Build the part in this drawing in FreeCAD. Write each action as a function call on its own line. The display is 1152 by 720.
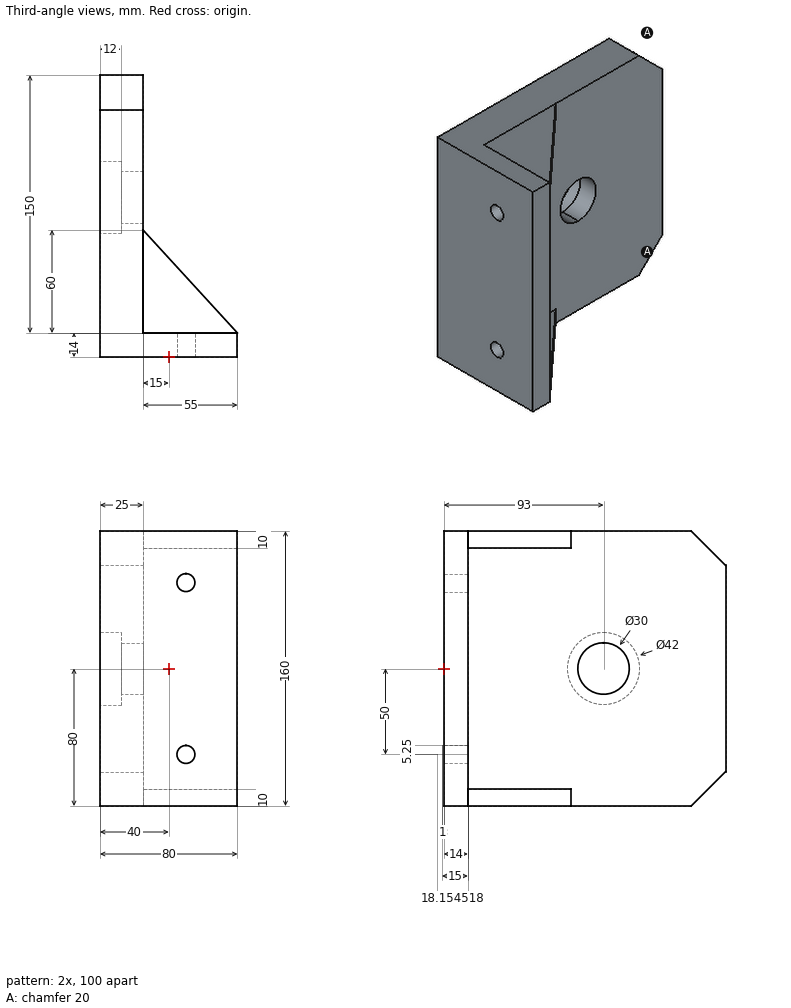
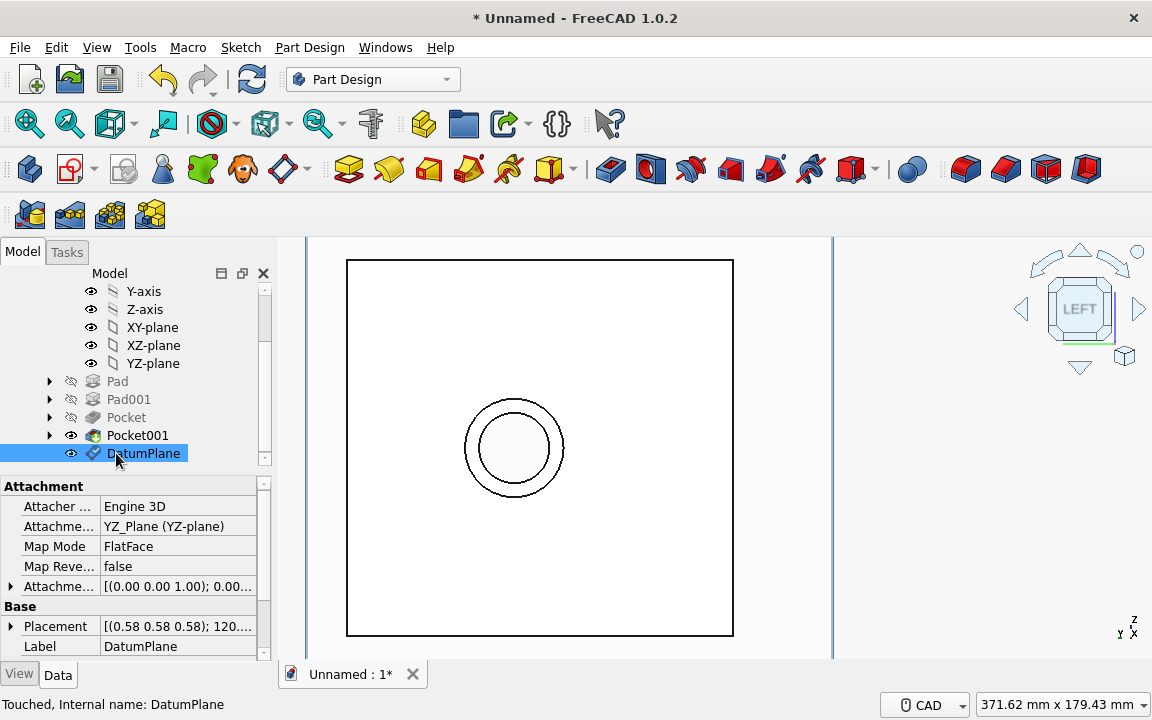
click(70, 170)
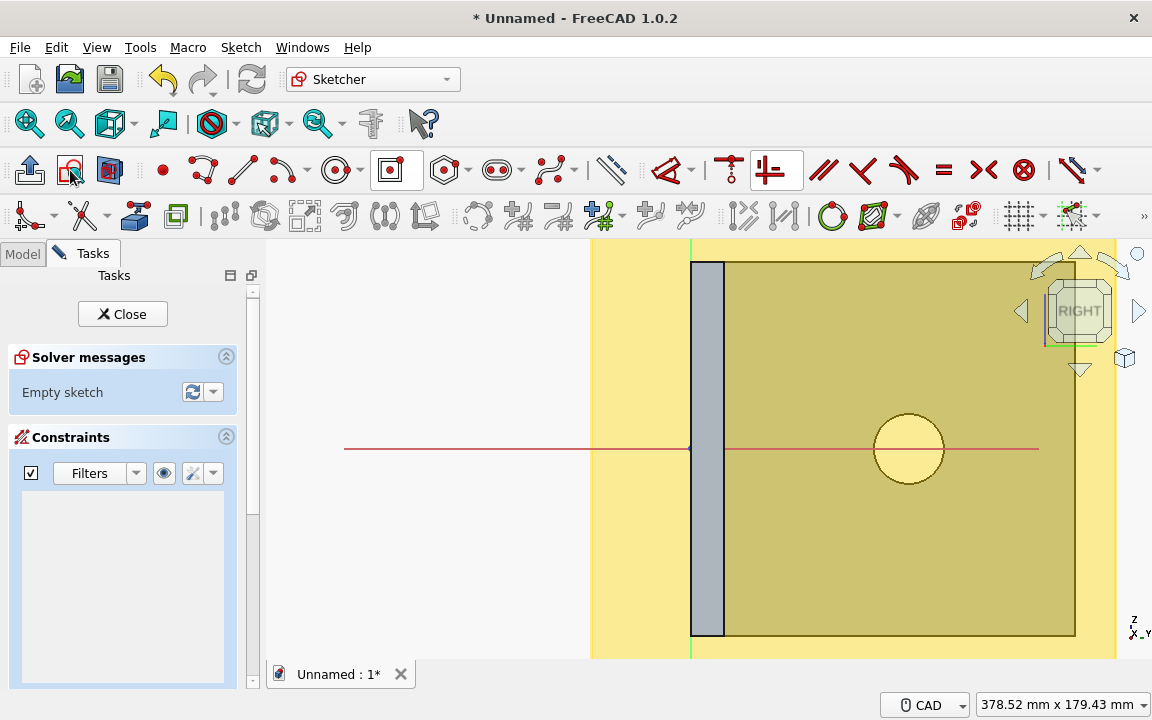
click(110, 170)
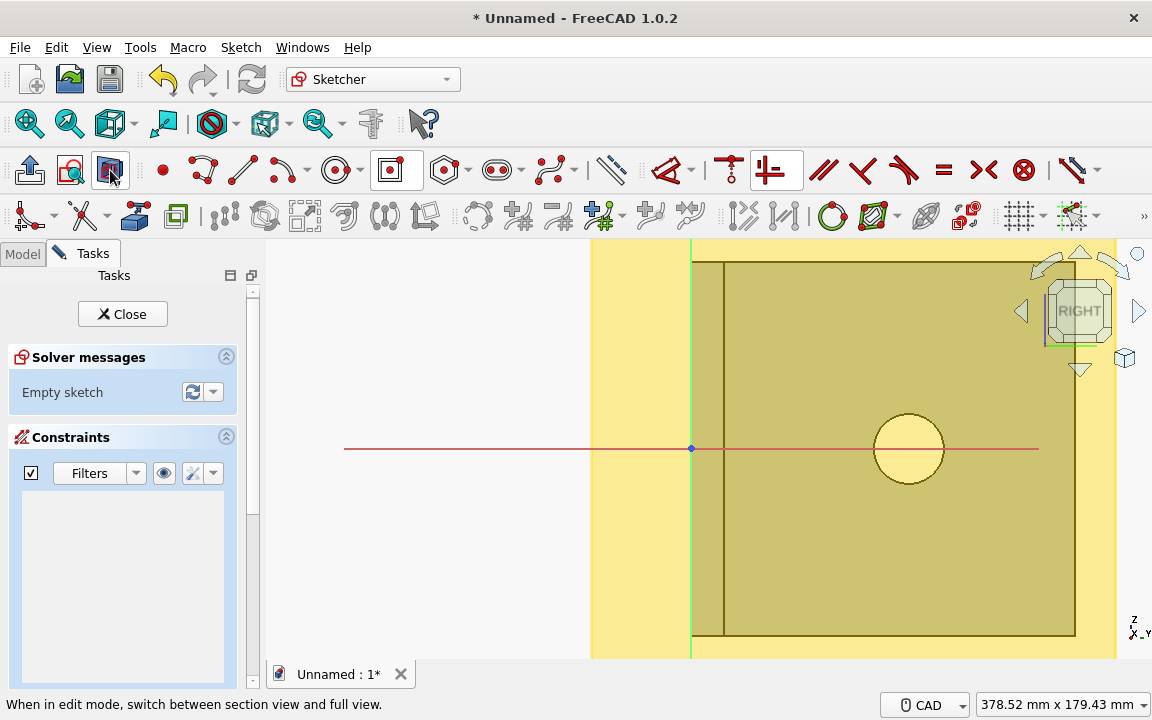
scroll(738, 555, up, 4)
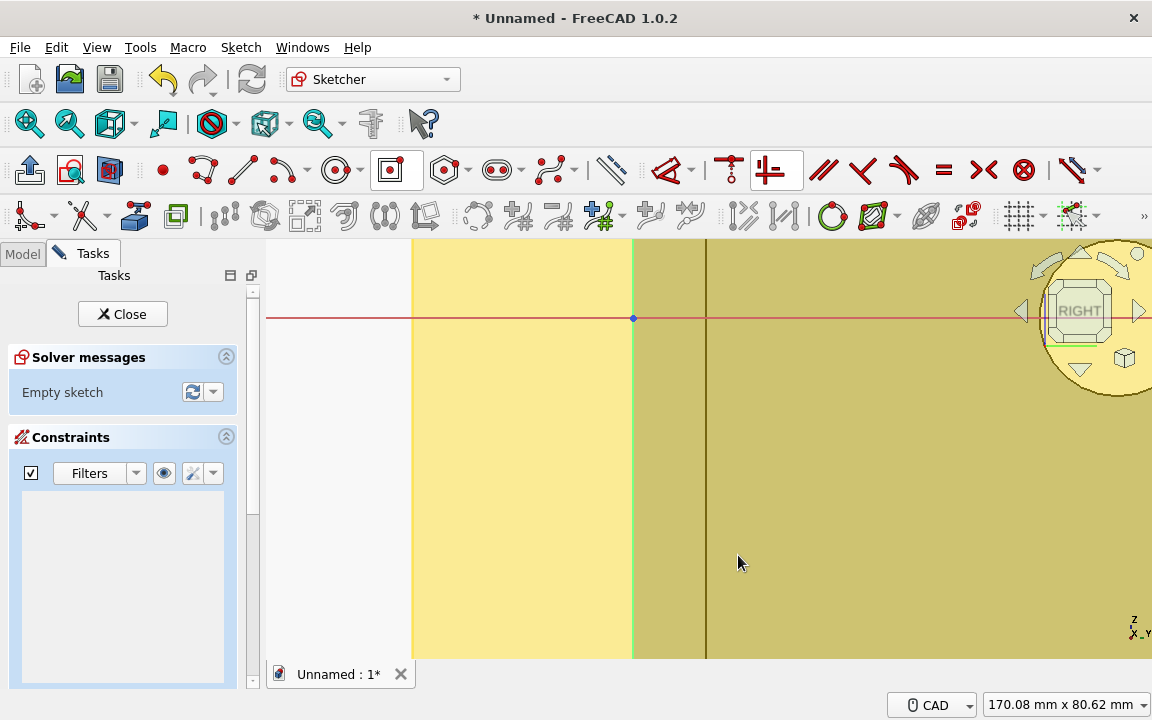
key(g)
key(m)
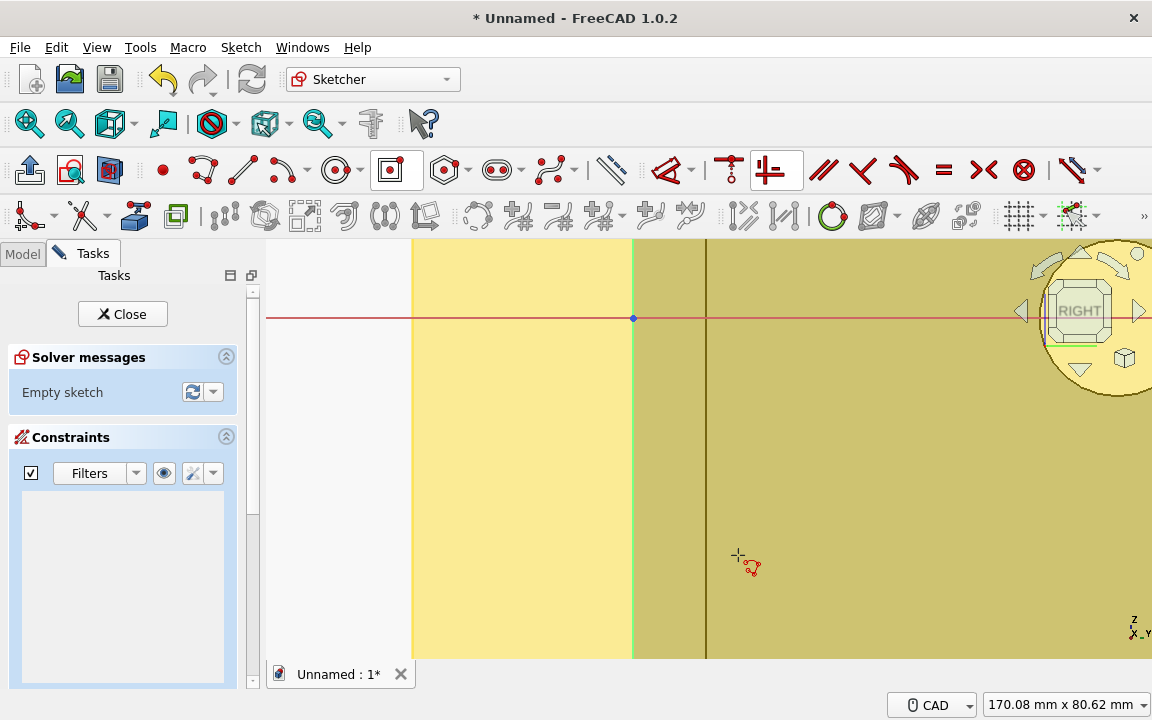
scroll(628, 551, up, 6)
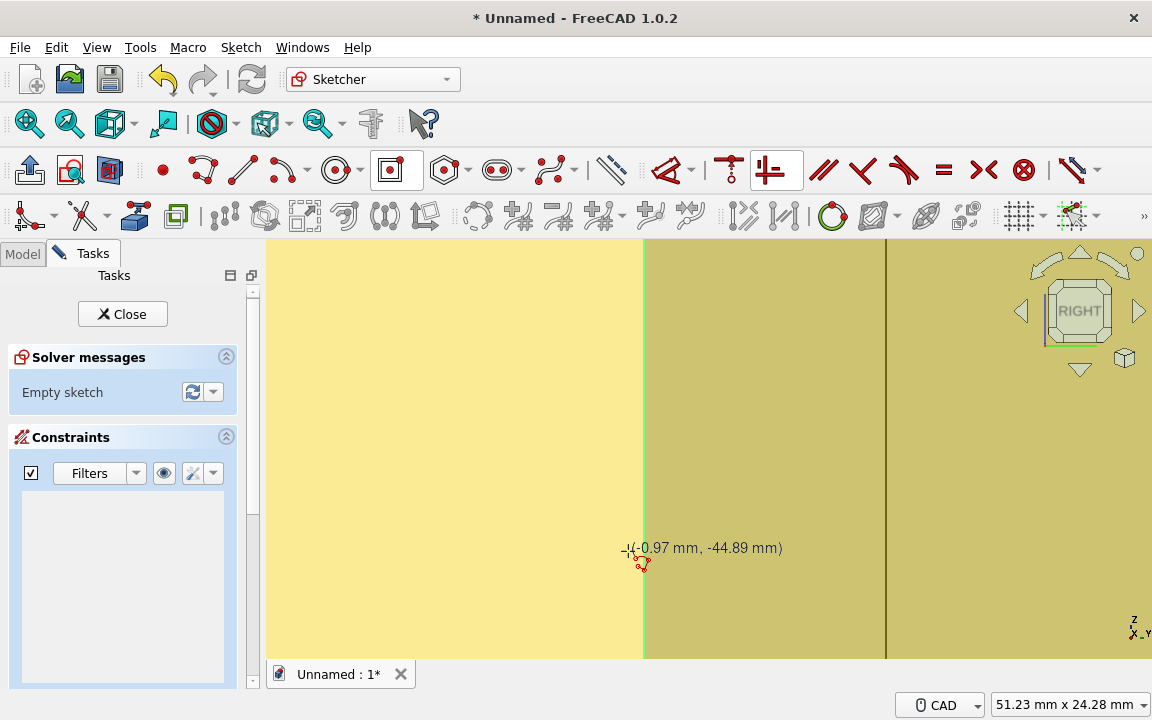
click(627, 550)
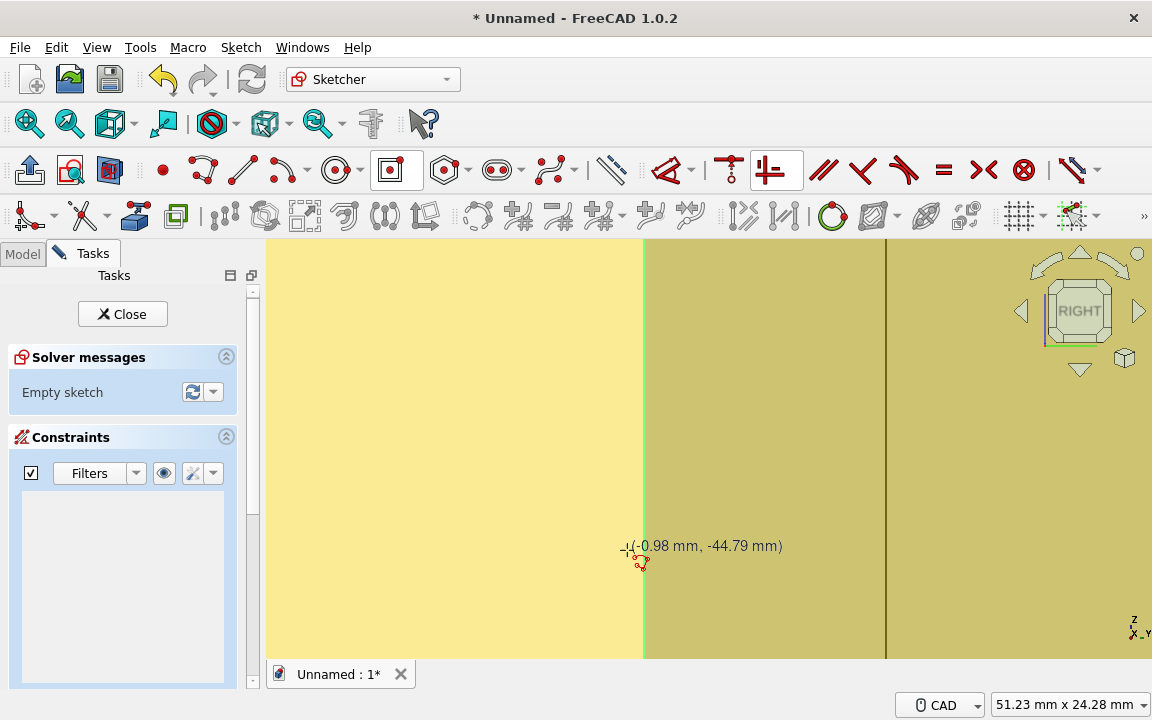
scroll(629, 553, down, 6)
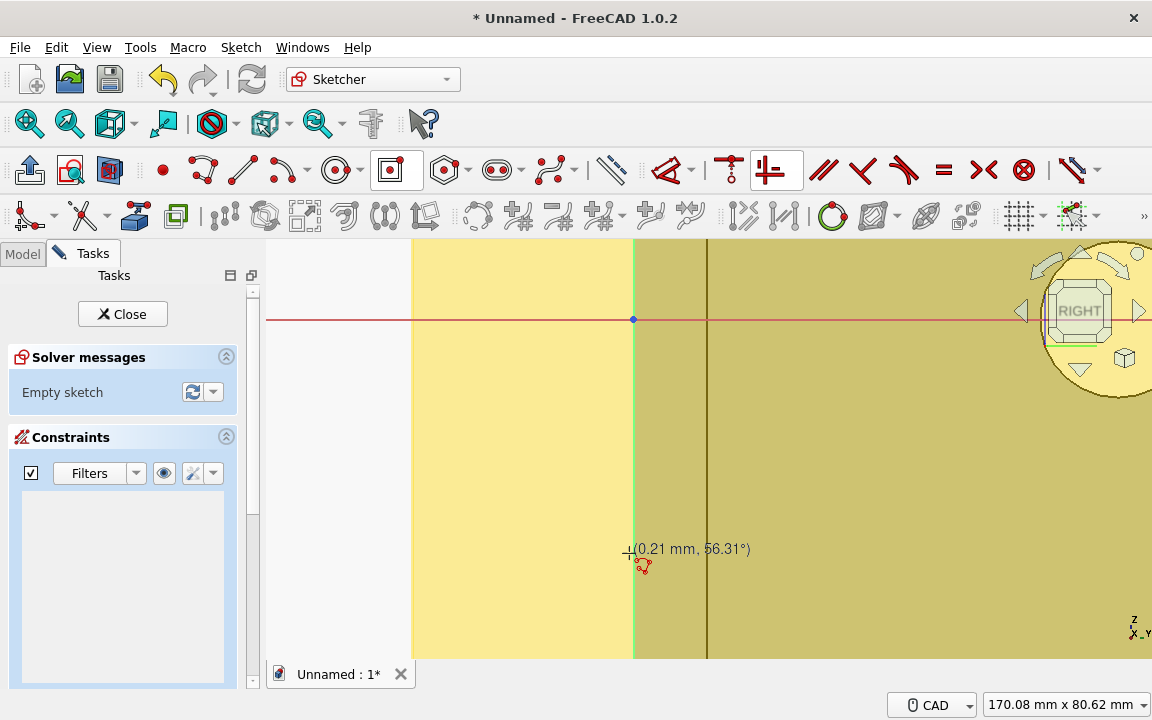
click(612, 580)
click(707, 580)
click(707, 553)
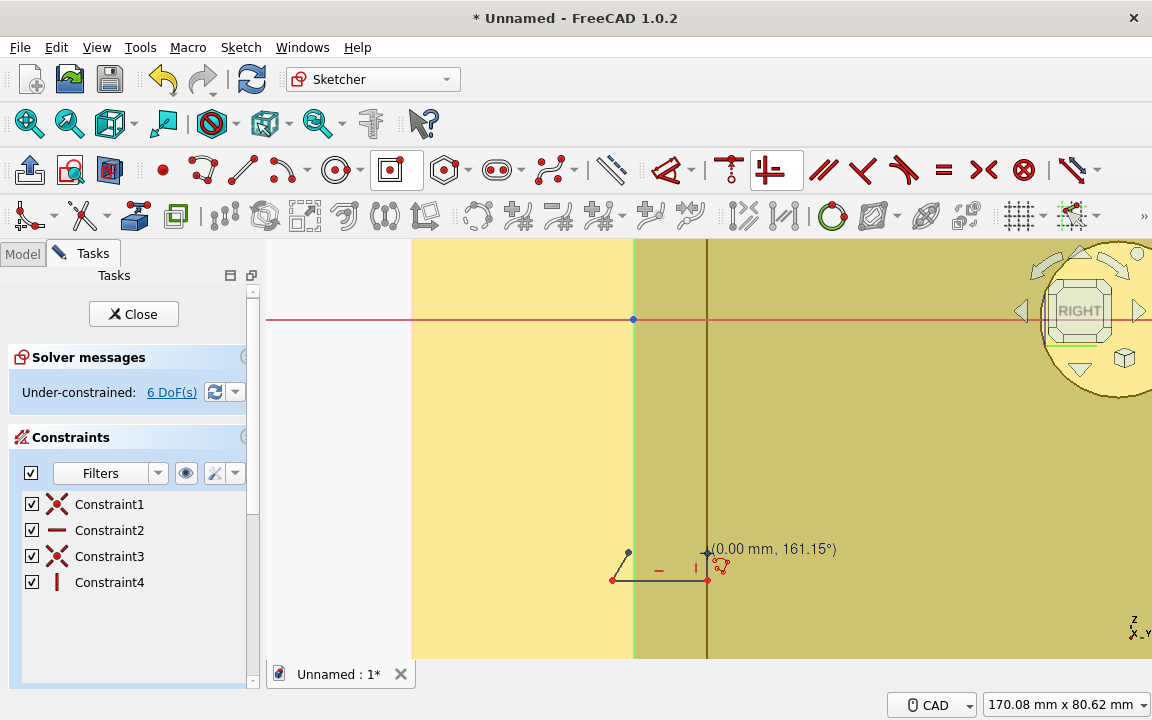
scroll(629, 553, up, 6)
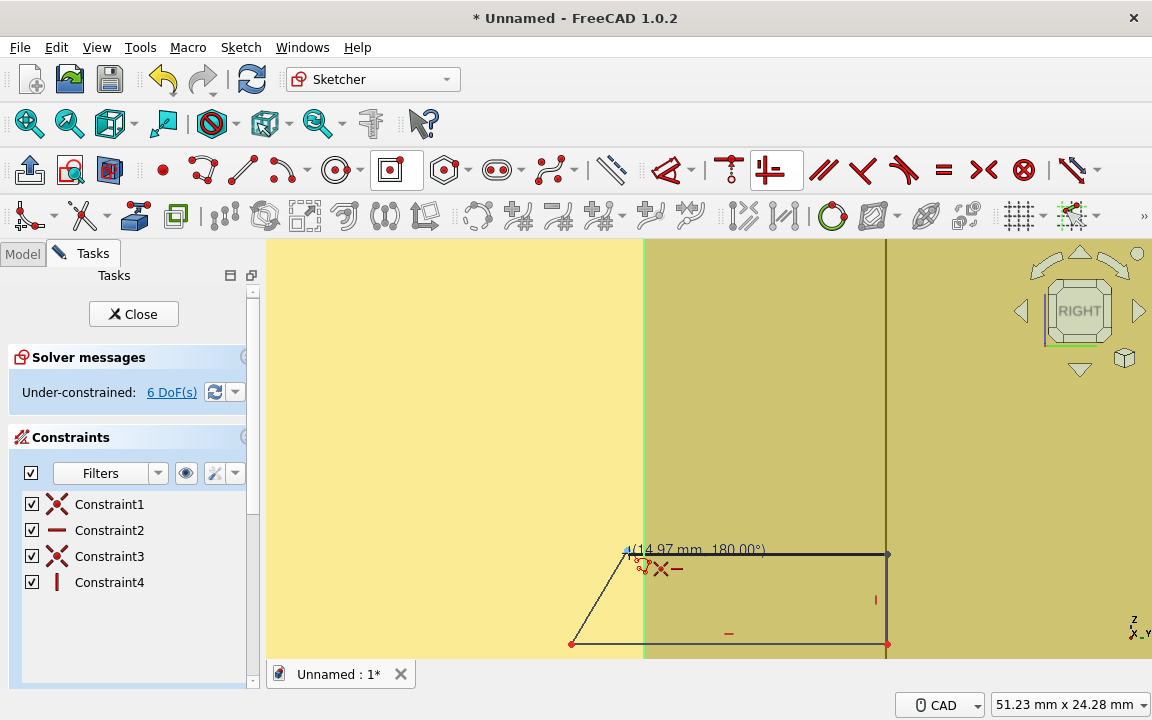
click(627, 551)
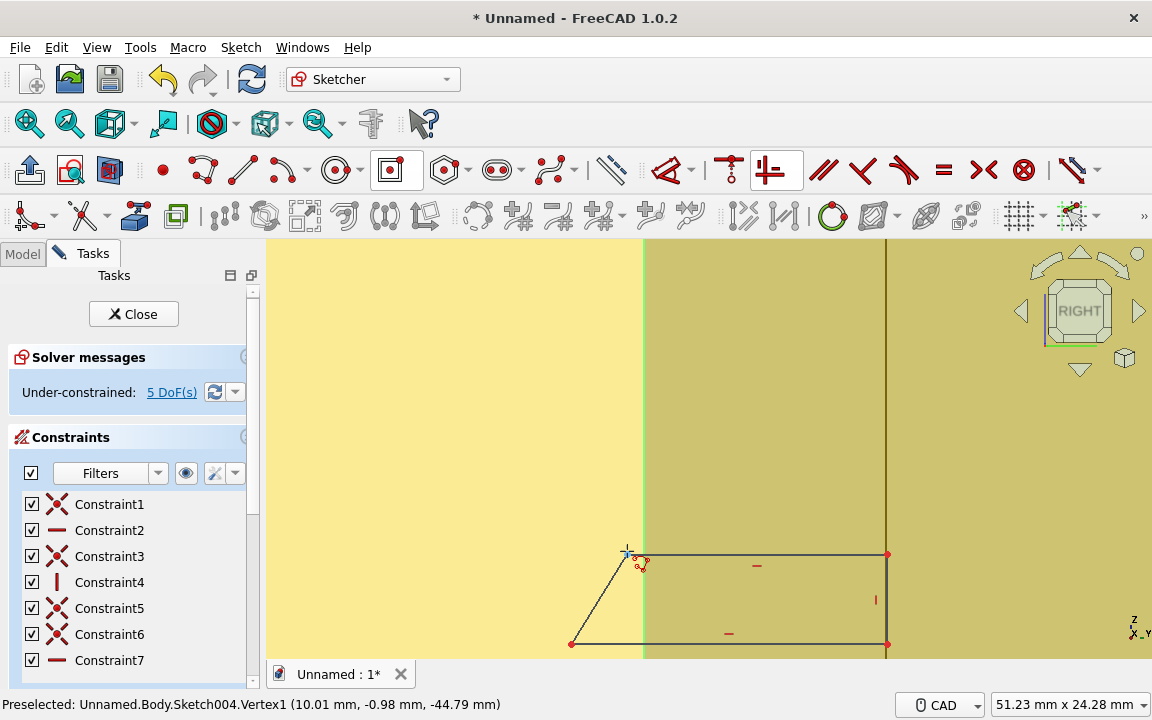
click(244, 170)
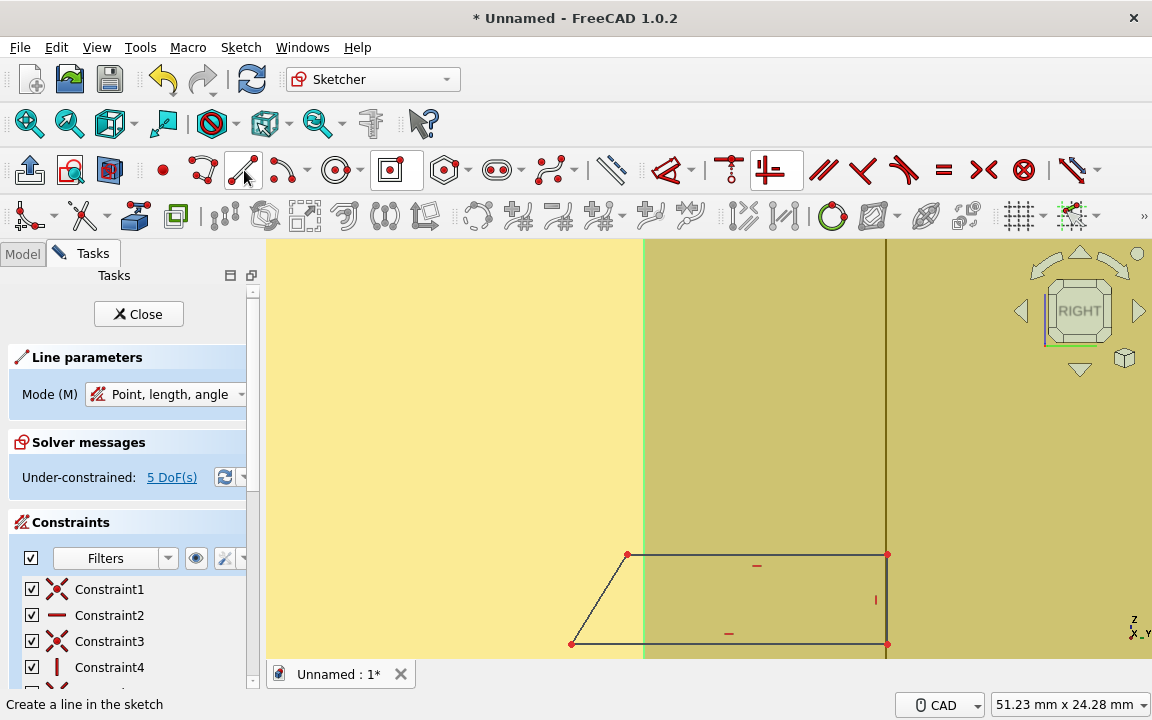
scroll(629, 553, down, 6)